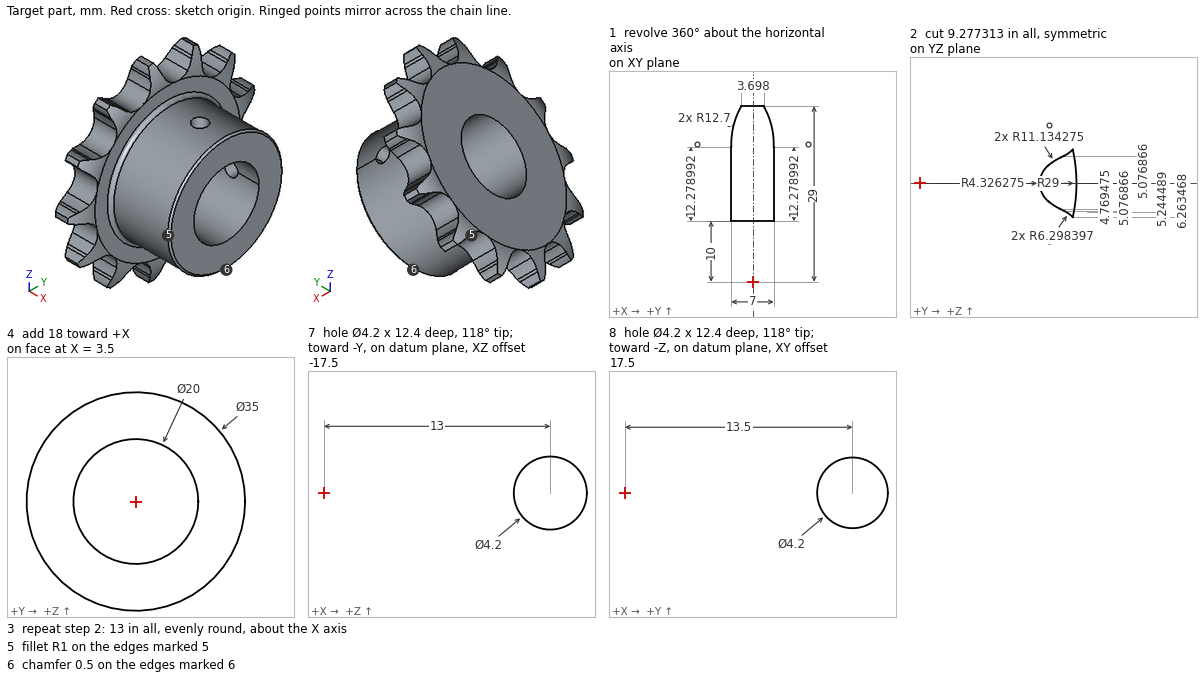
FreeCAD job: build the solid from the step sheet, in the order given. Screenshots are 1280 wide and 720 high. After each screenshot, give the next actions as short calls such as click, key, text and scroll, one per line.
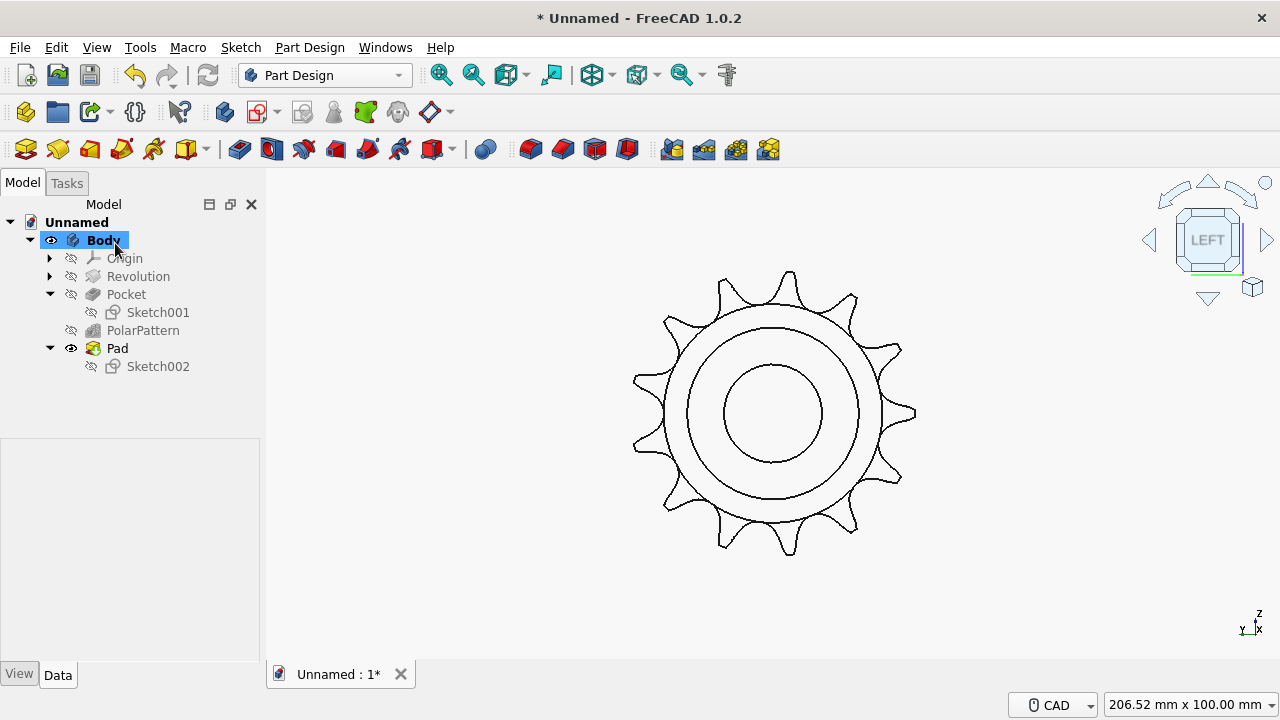
key(0)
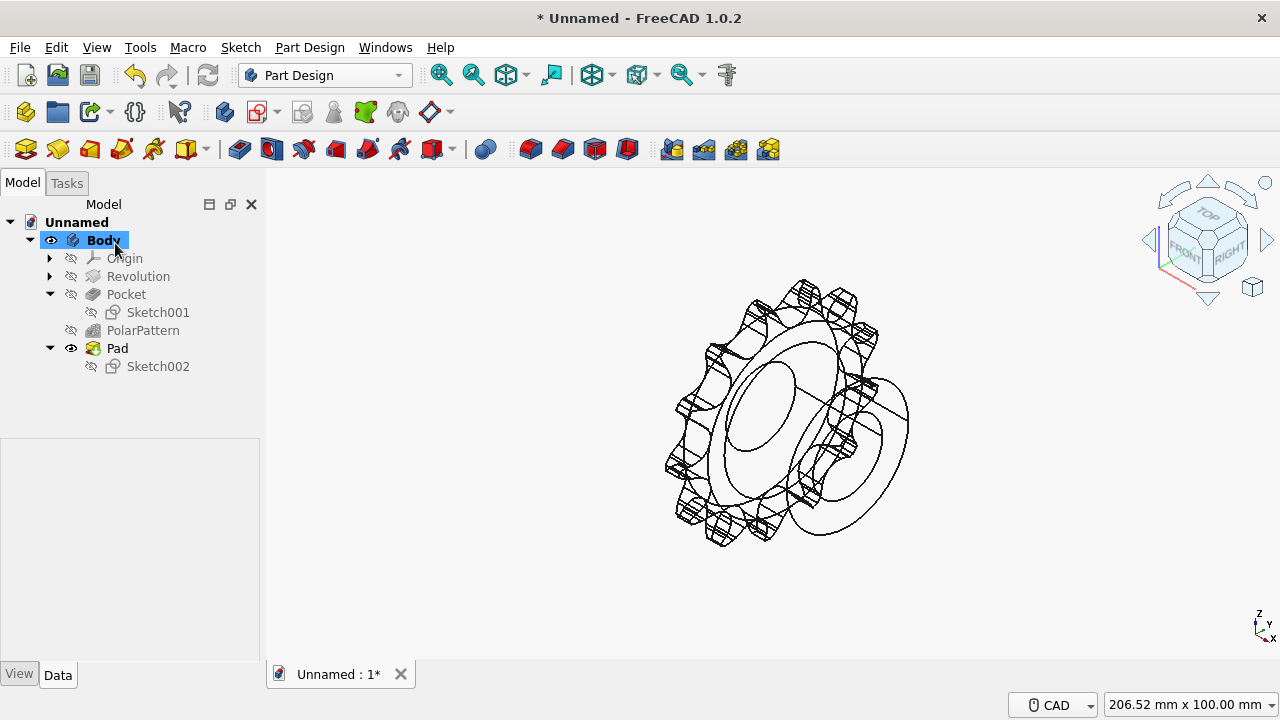
click(724, 455)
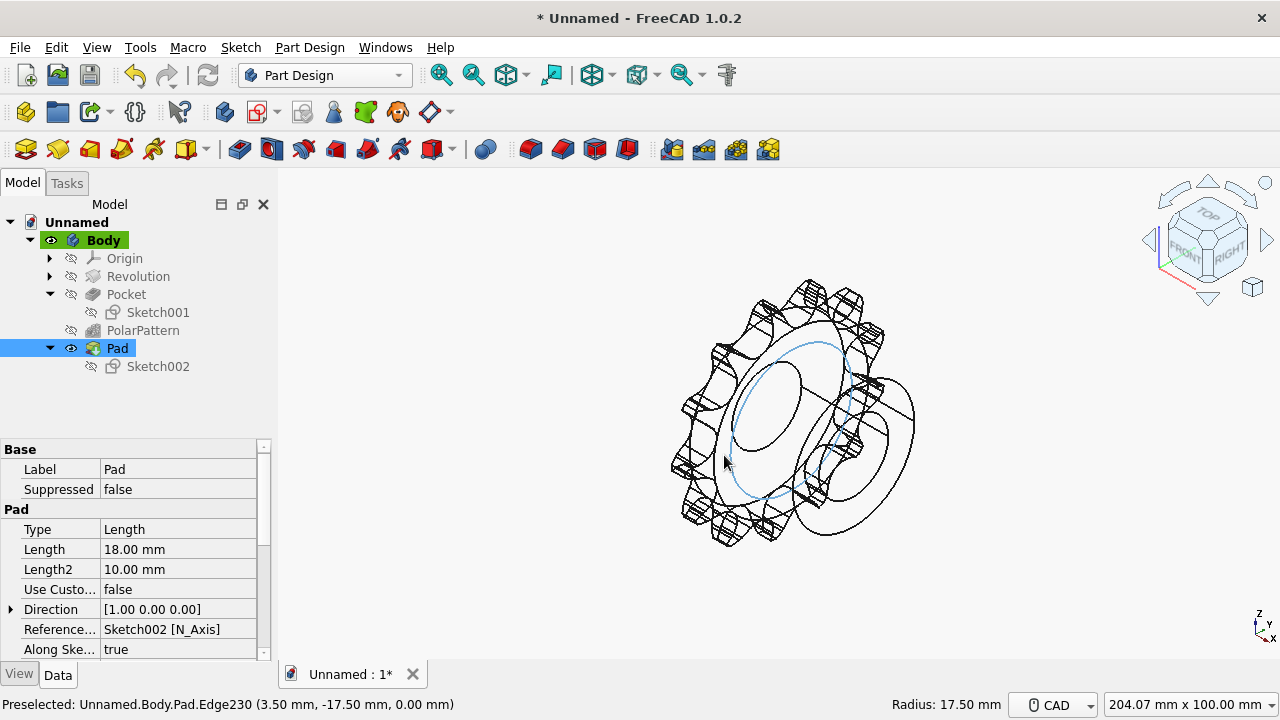
key(v)
key(1)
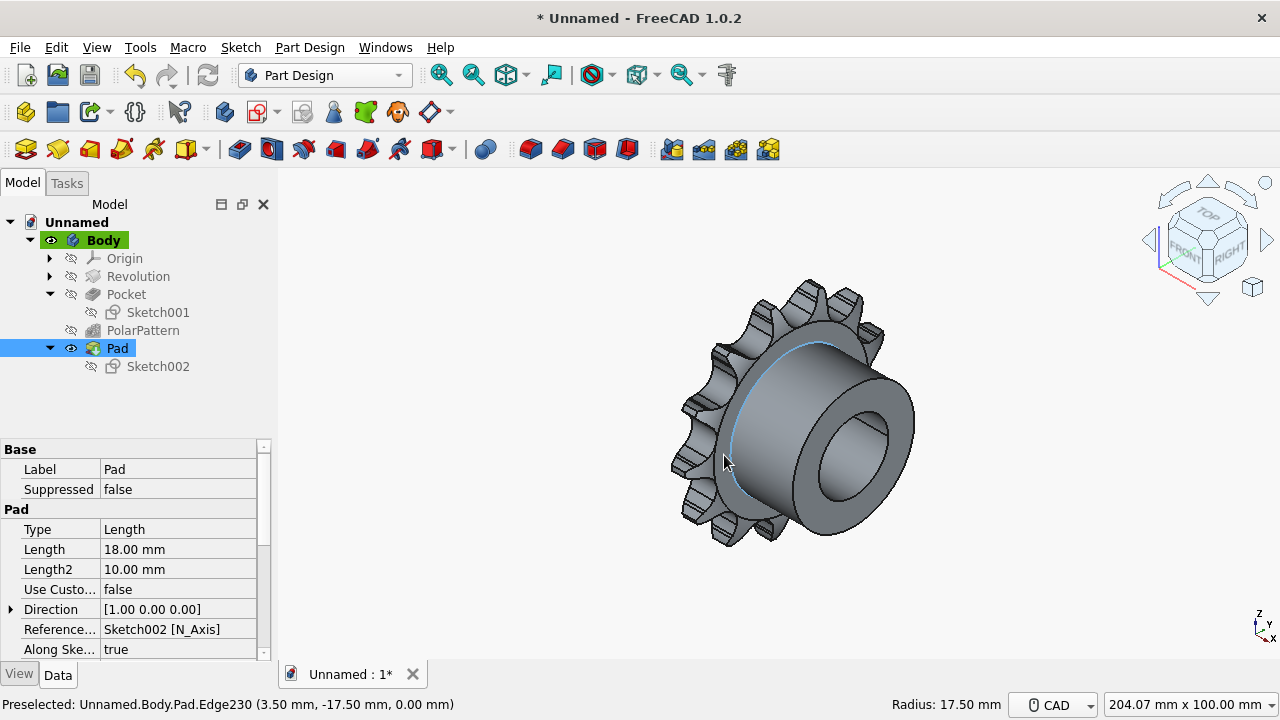
click(532, 150)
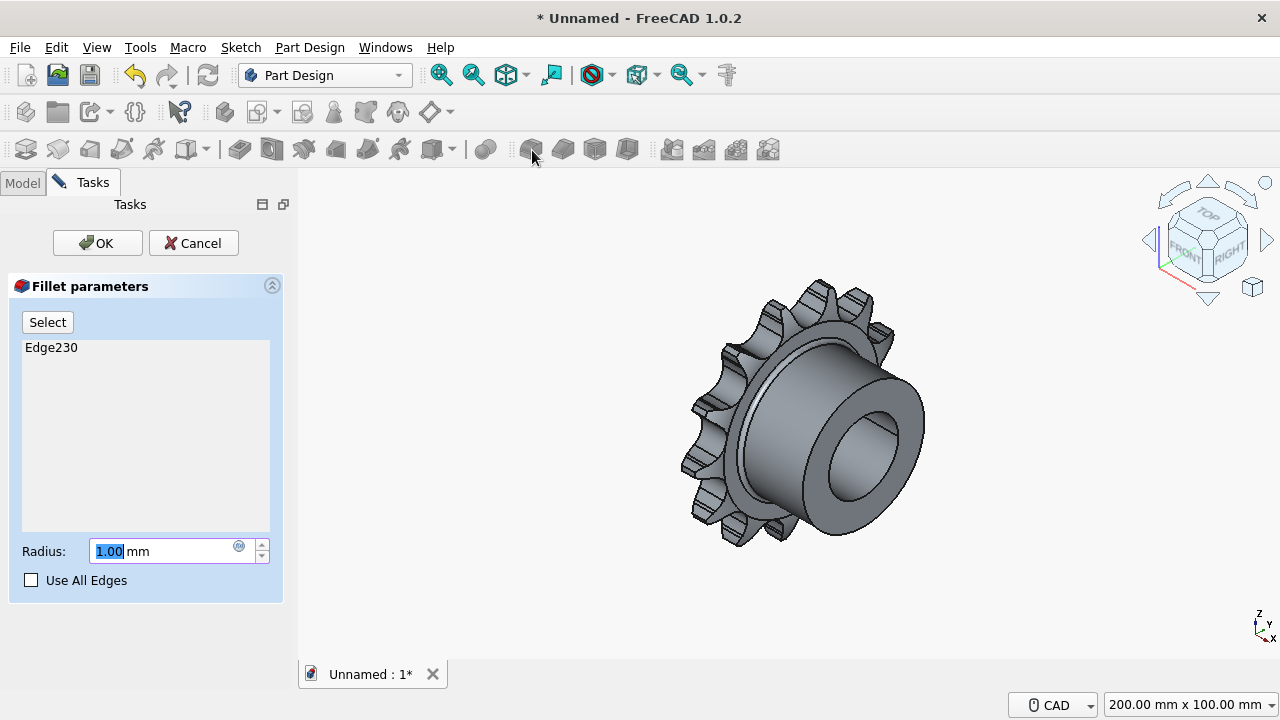
text(1)
key(Tab)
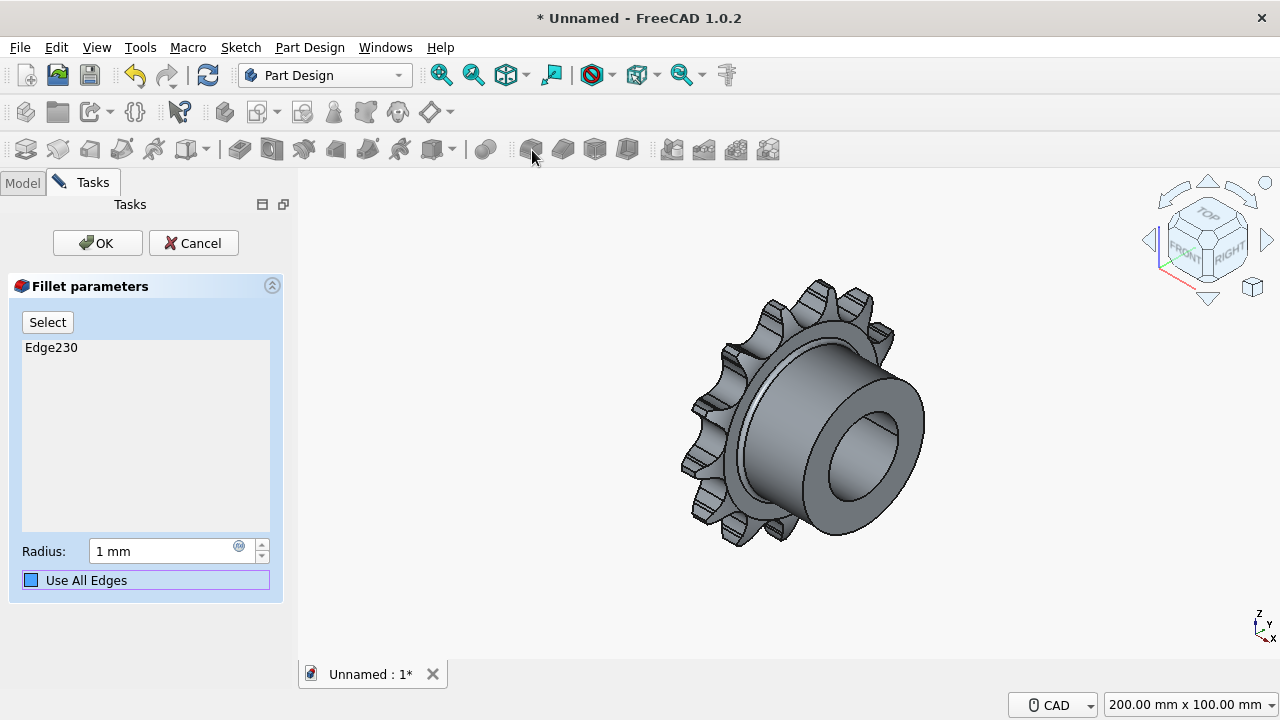
click(98, 243)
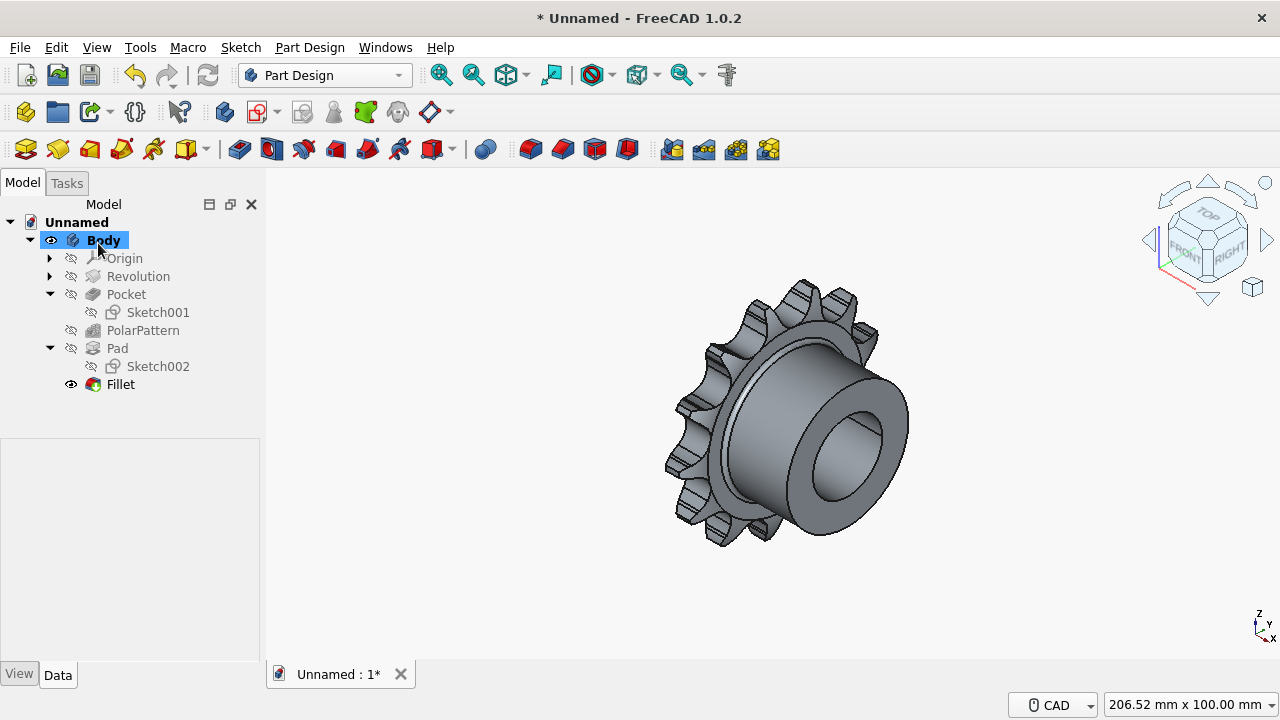
click(787, 491)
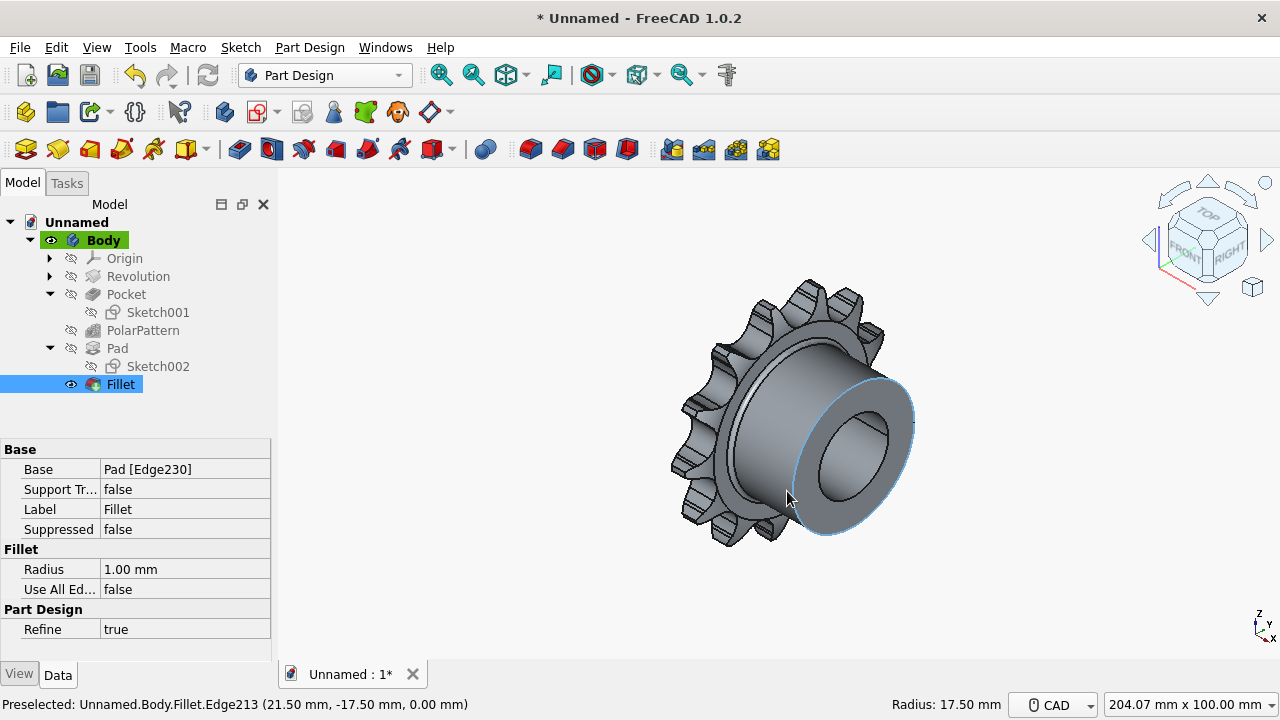
click(564, 150)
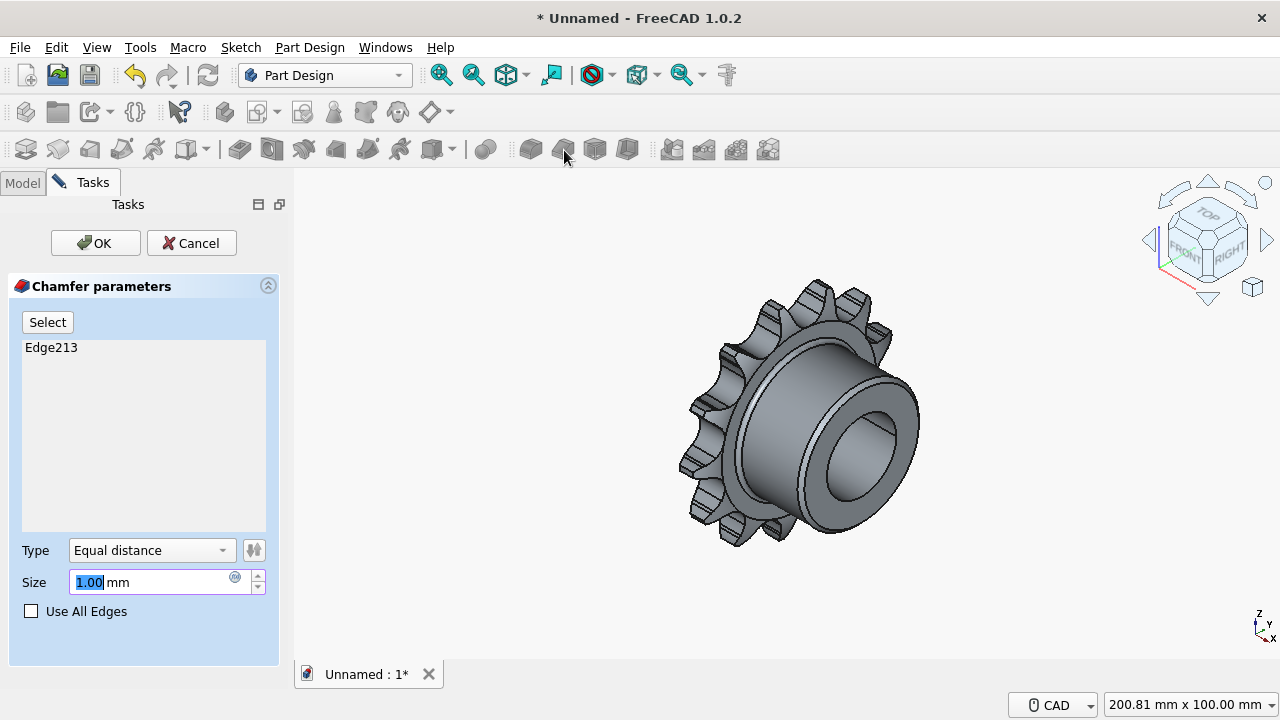
text(0.5)
key(Tab)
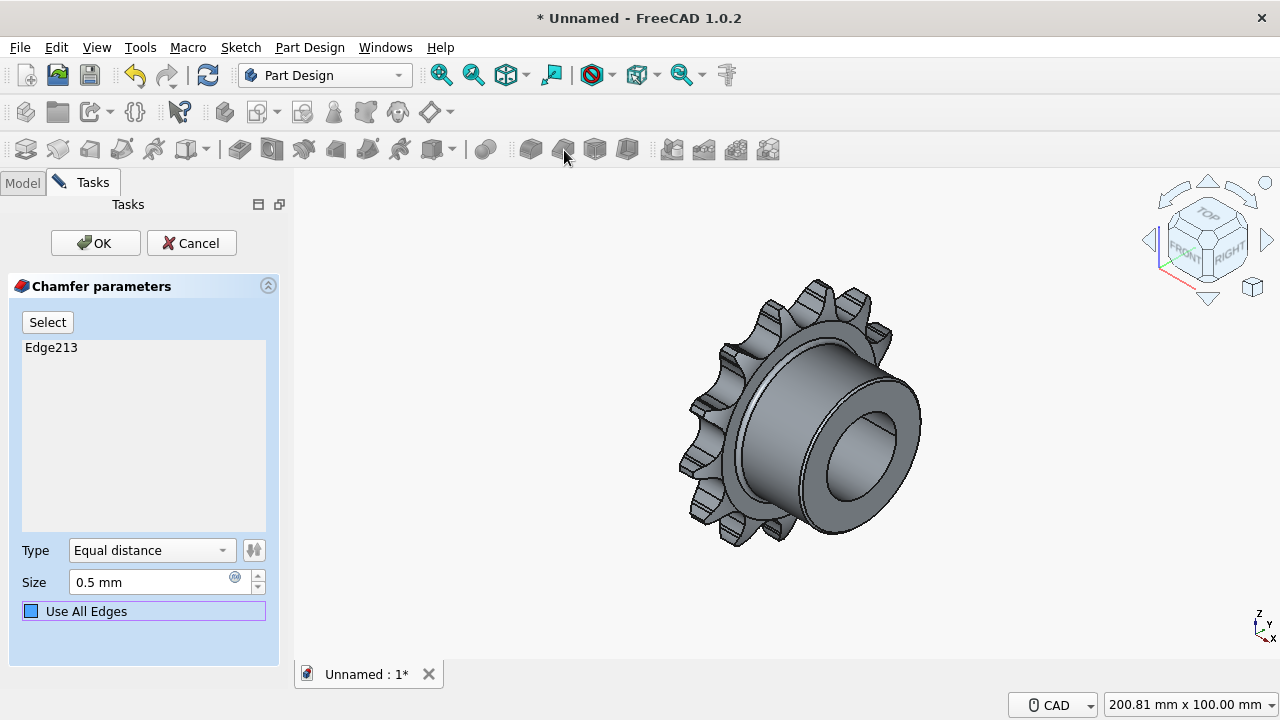
click(96, 243)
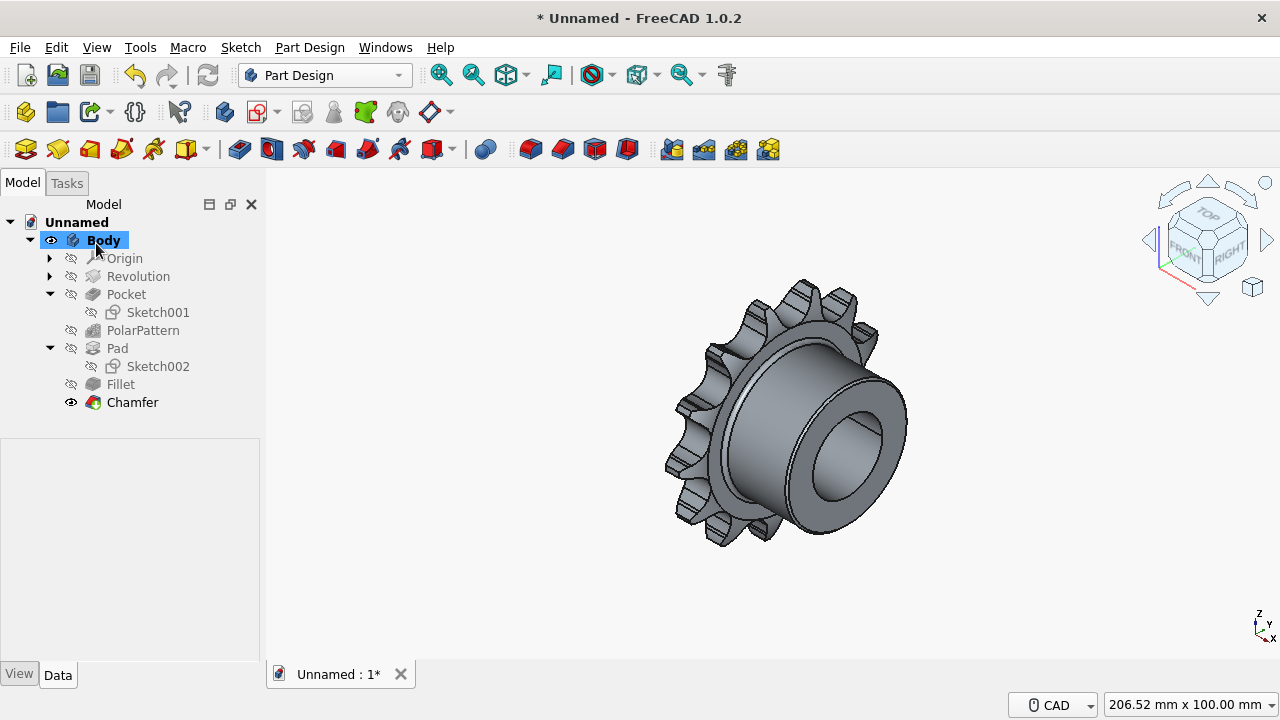
click(50, 258)